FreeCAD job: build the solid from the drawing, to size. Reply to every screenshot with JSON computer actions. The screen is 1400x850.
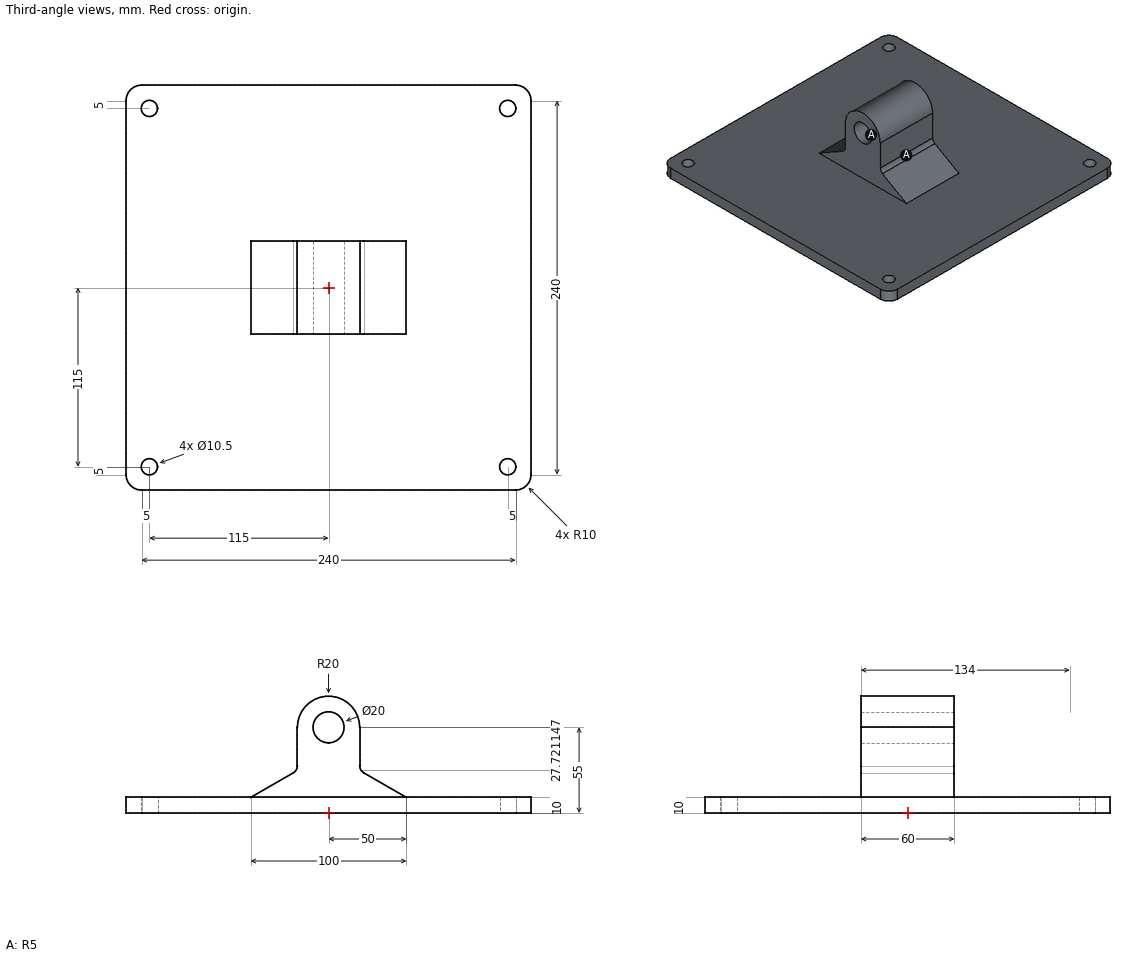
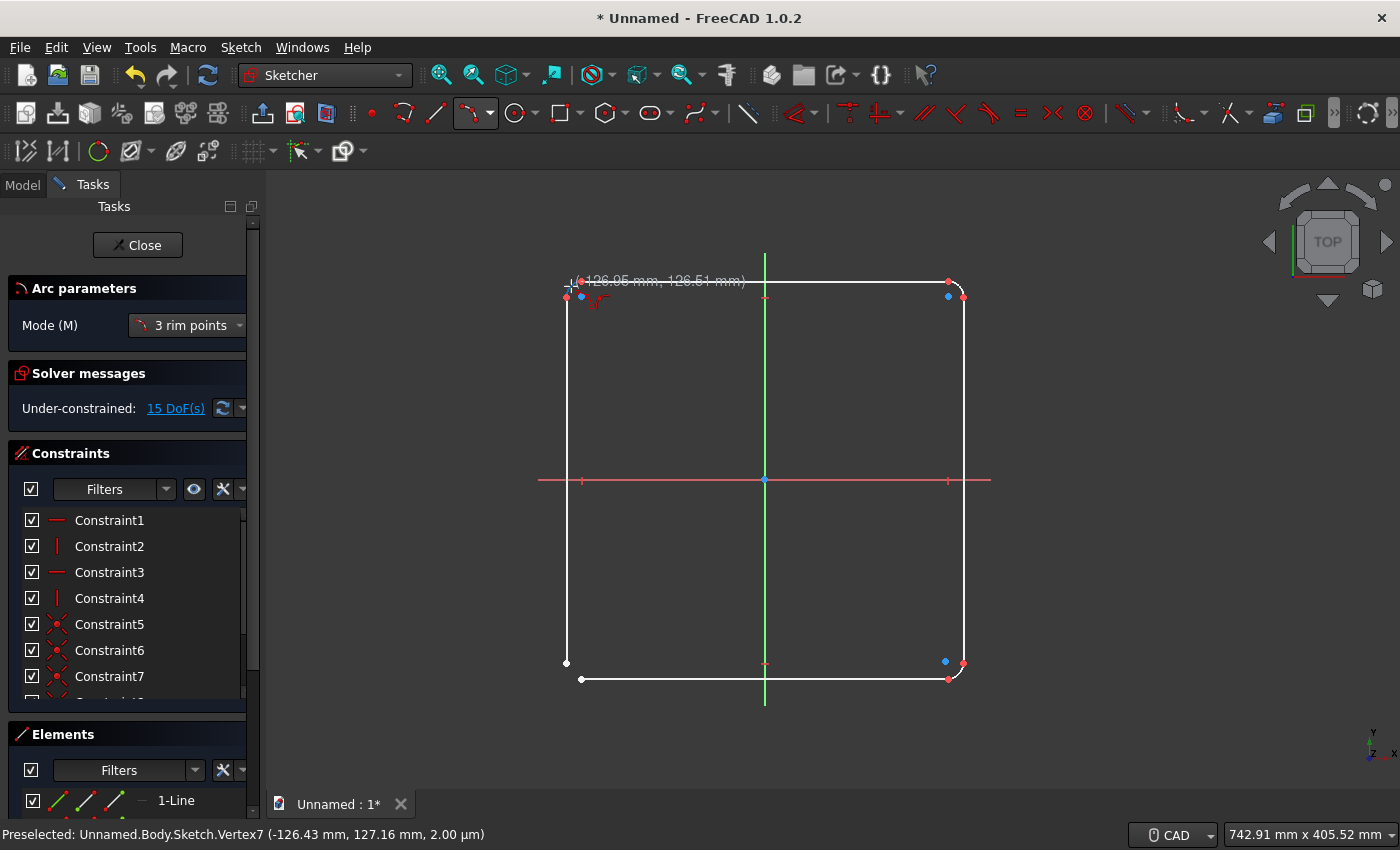
{"action": "left_click", "coordinate": [567, 663]}
{"action": "left_click", "coordinate": [582, 679]}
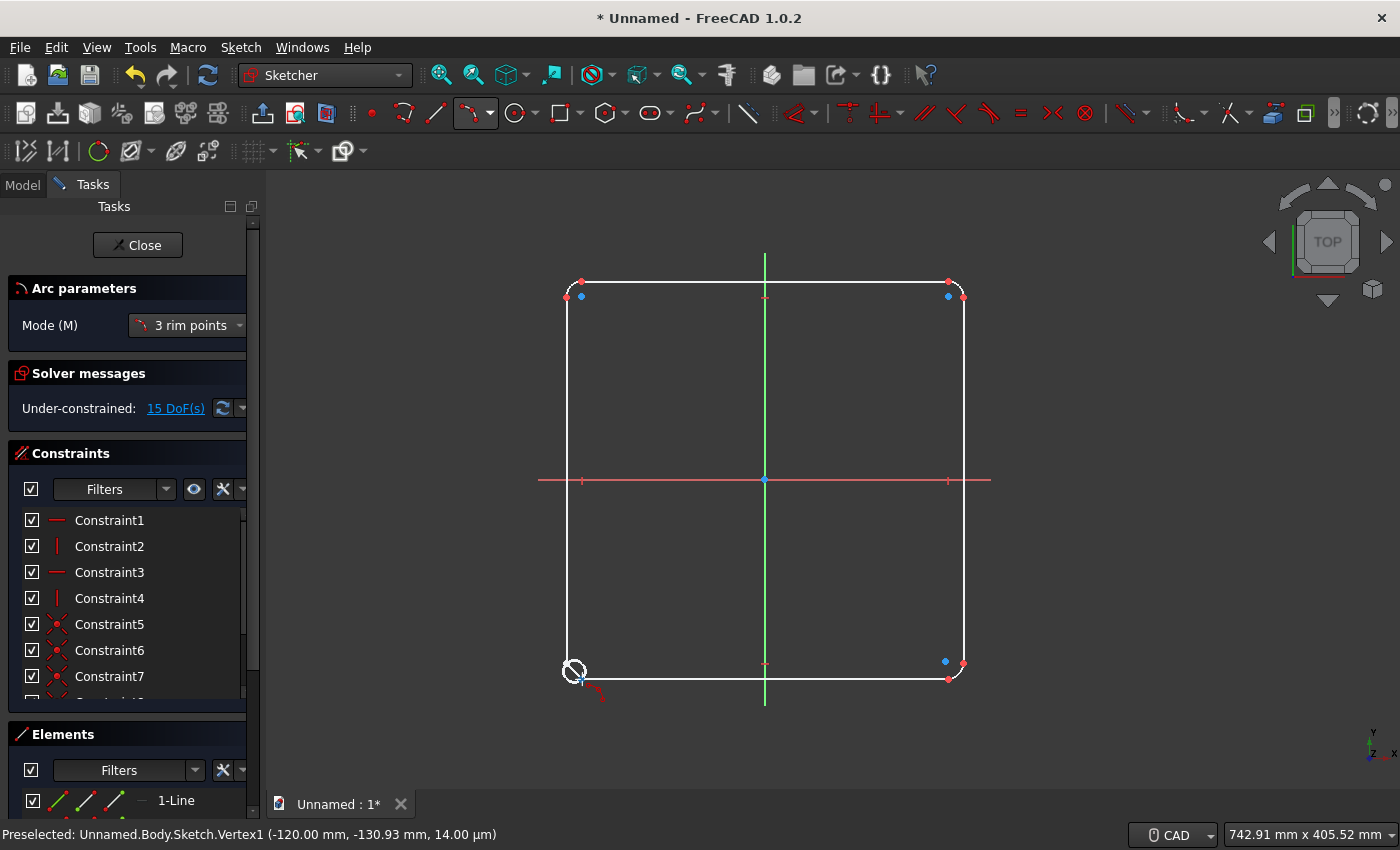
{"action": "scroll", "coordinate": [571, 673], "scroll_direction": "up", "scroll_amount": 7}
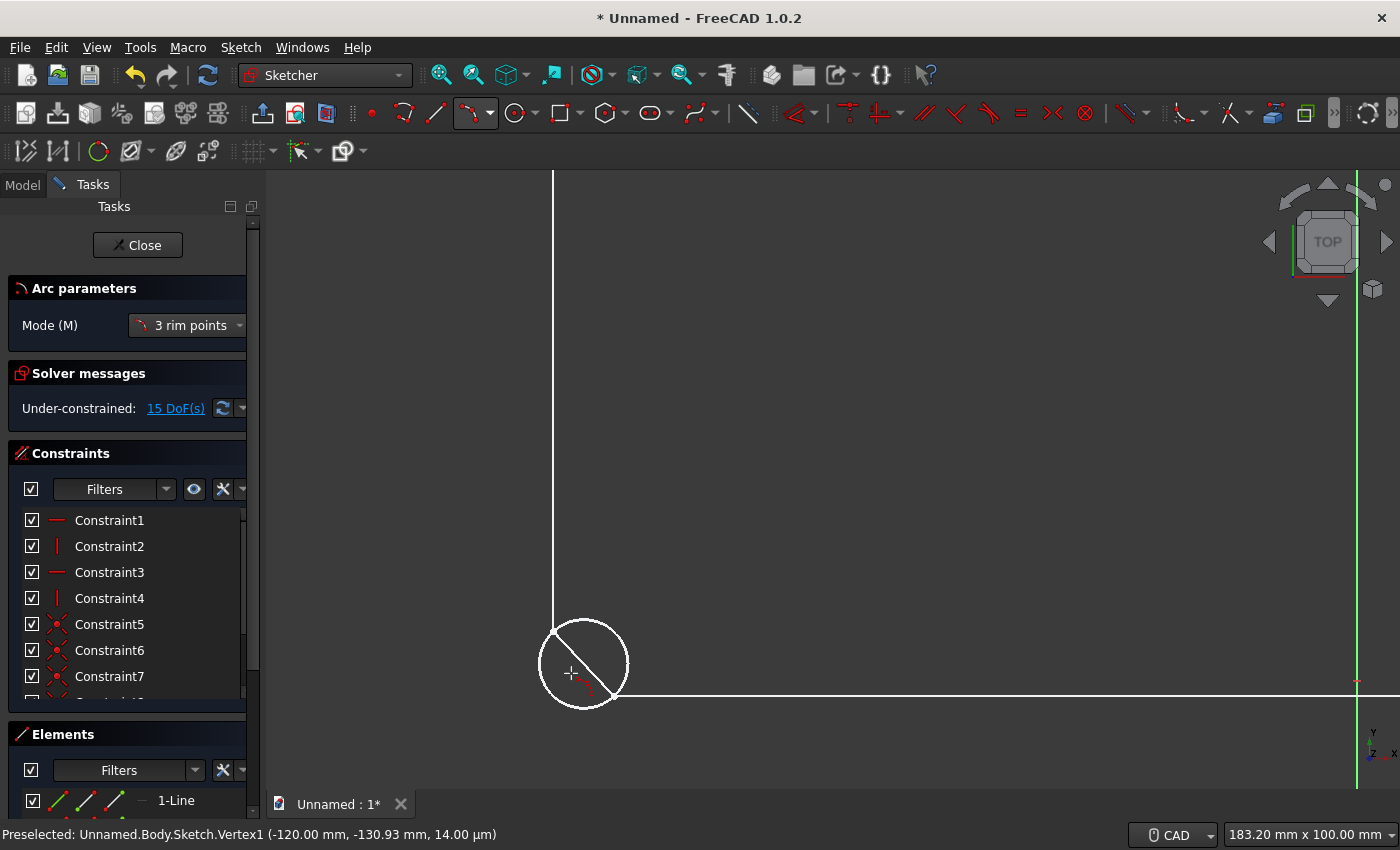
{"action": "left_click", "coordinate": [570, 672]}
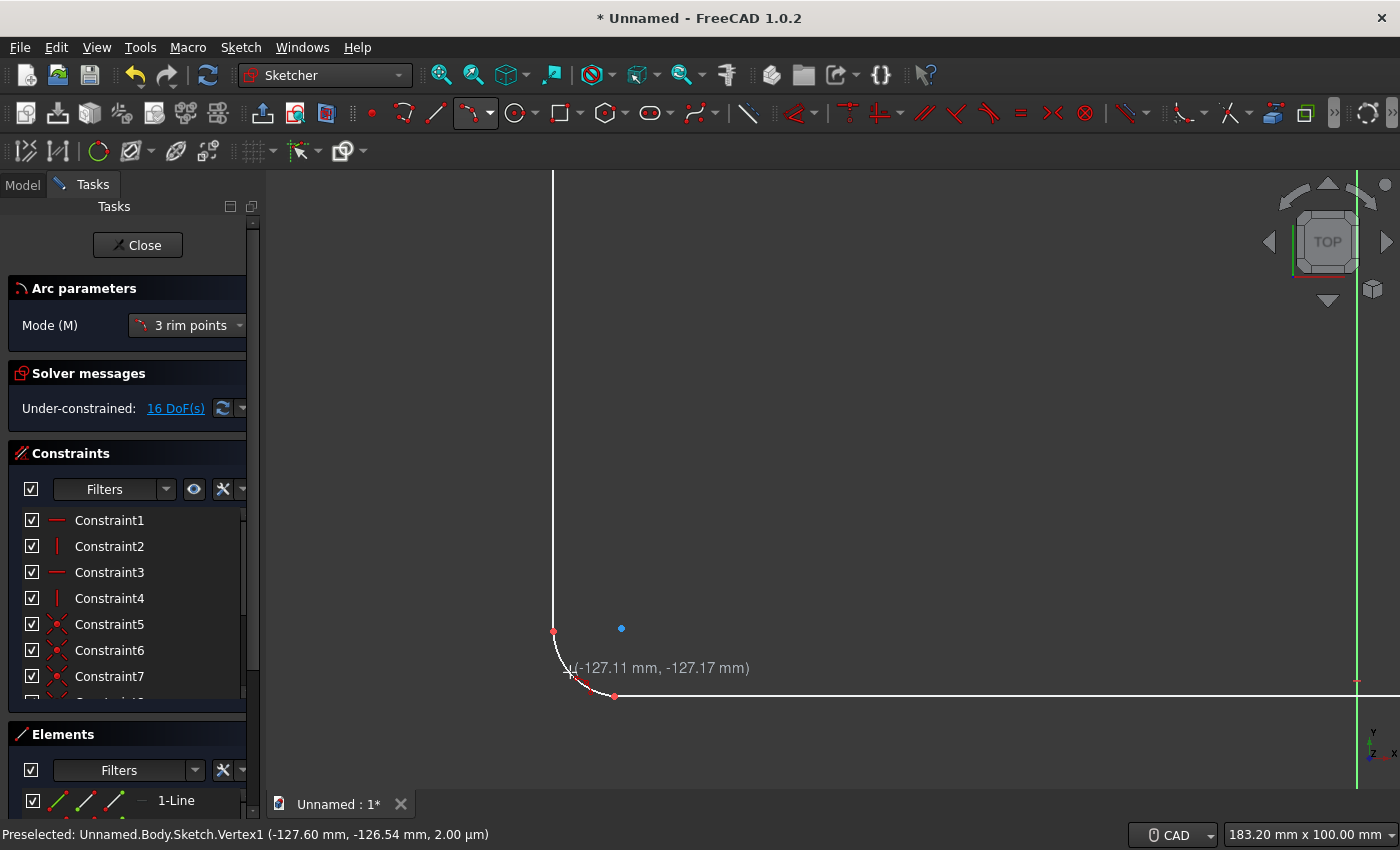
{"action": "left_click", "coordinate": [516, 114]}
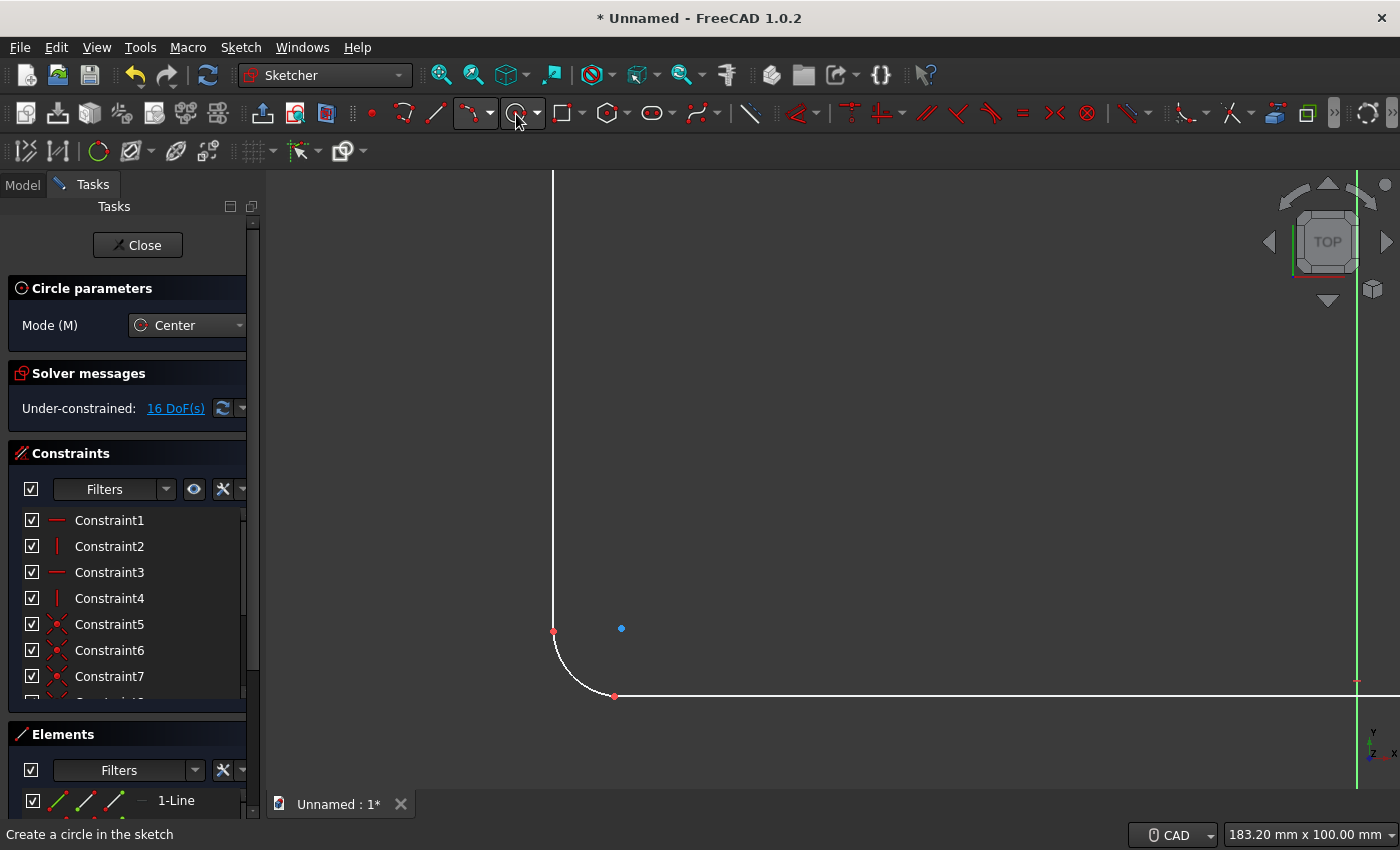
{"action": "left_click", "coordinate": [645, 598]}
{"action": "left_click", "coordinate": [668, 575]}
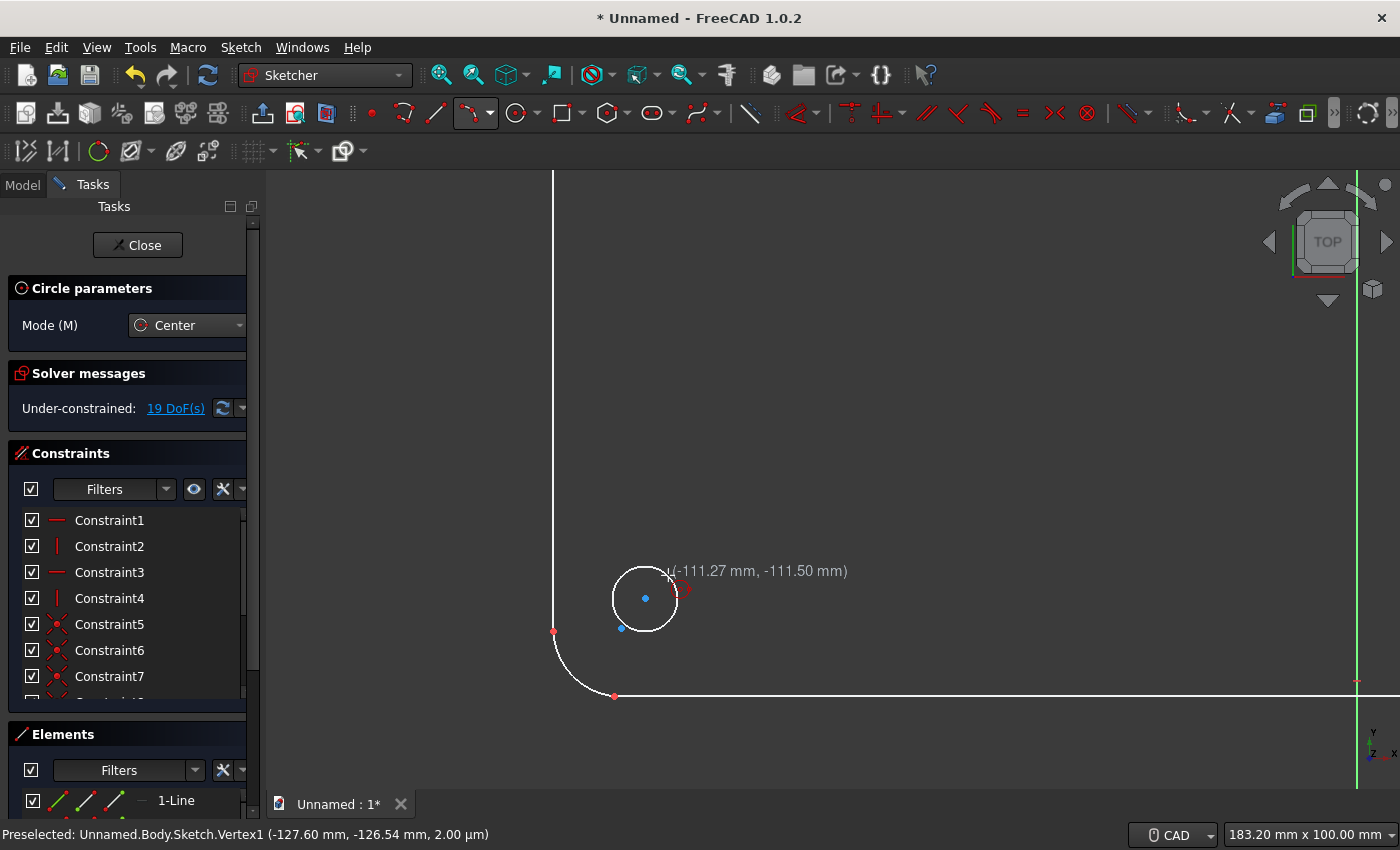
{"action": "scroll", "coordinate": [571, 674], "scroll_direction": "down", "scroll_amount": 7}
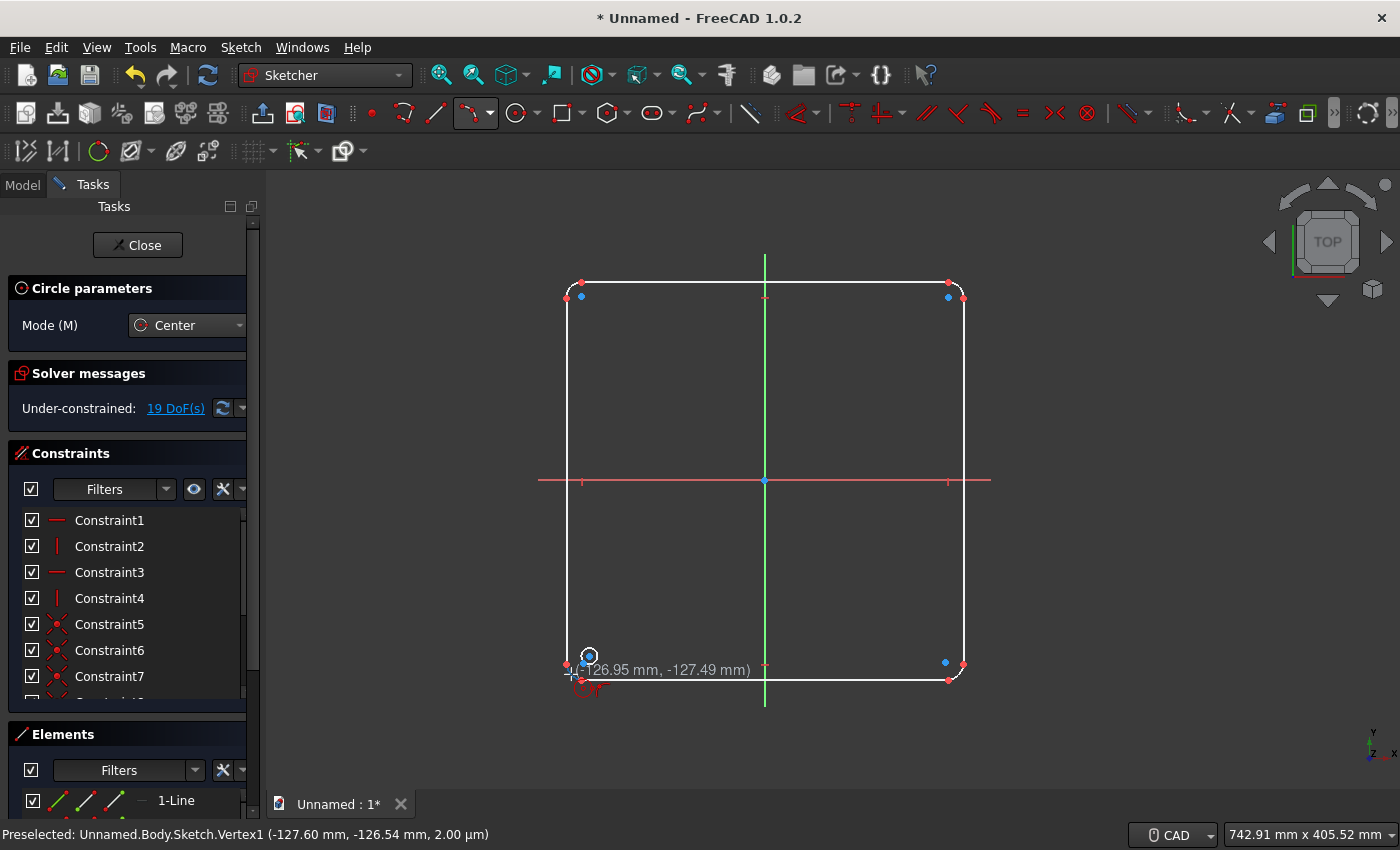
{"action": "scroll", "coordinate": [941, 656], "scroll_direction": "up", "scroll_amount": 6}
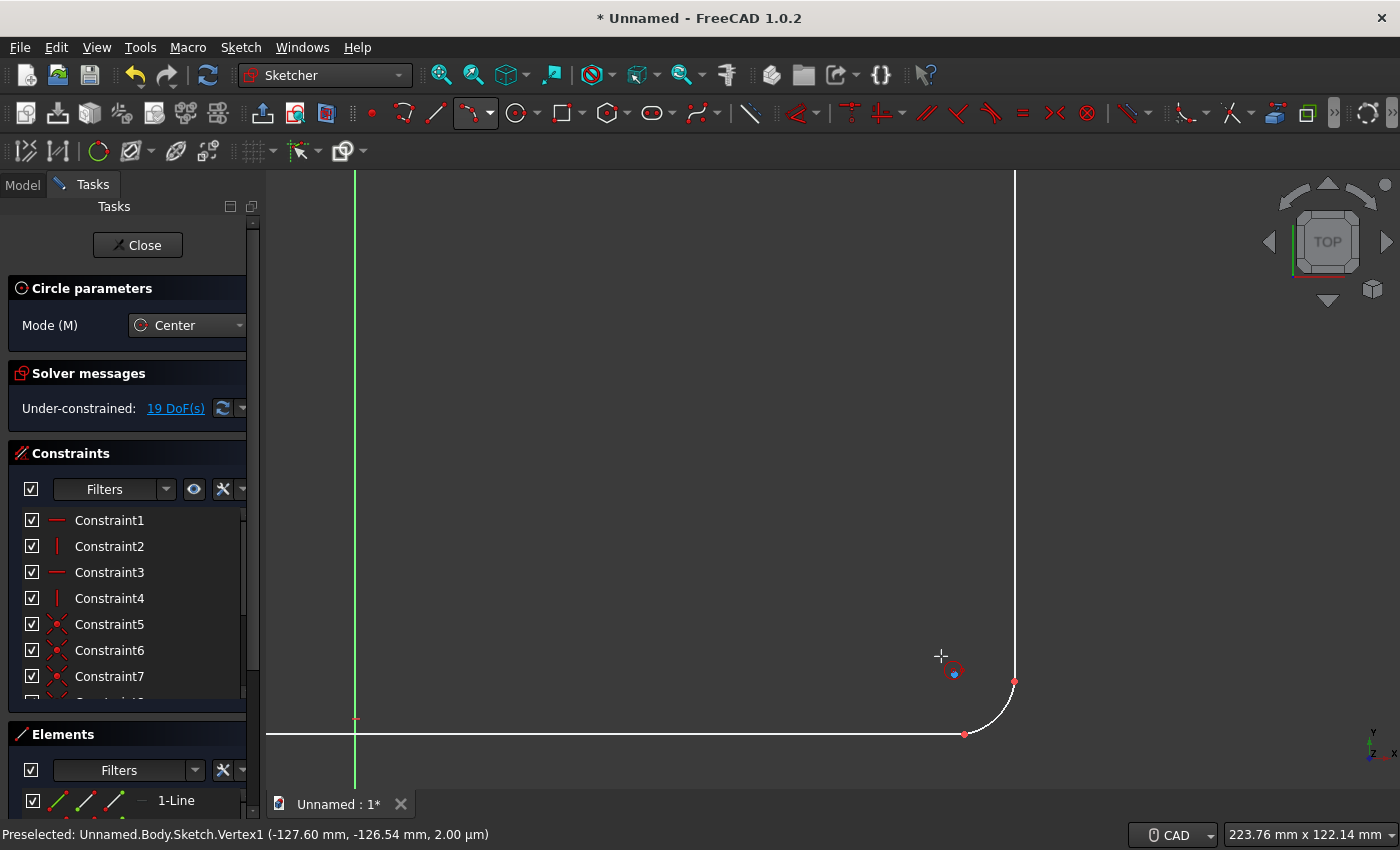
{"action": "left_click", "coordinate": [938, 653]}
{"action": "left_click", "coordinate": [957, 635]}